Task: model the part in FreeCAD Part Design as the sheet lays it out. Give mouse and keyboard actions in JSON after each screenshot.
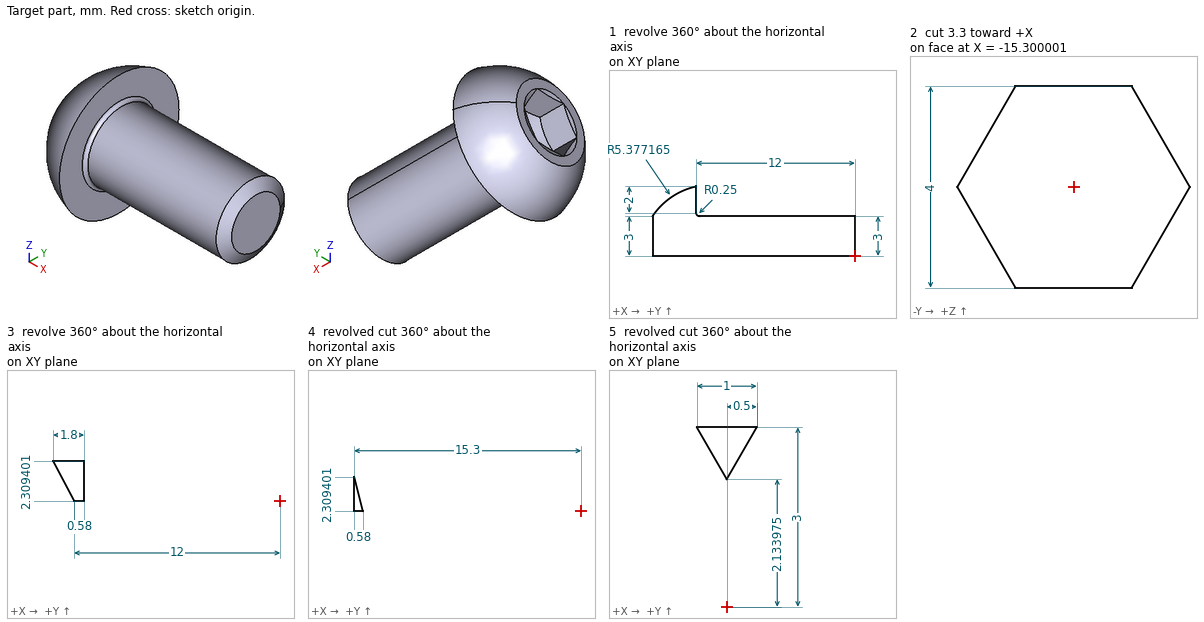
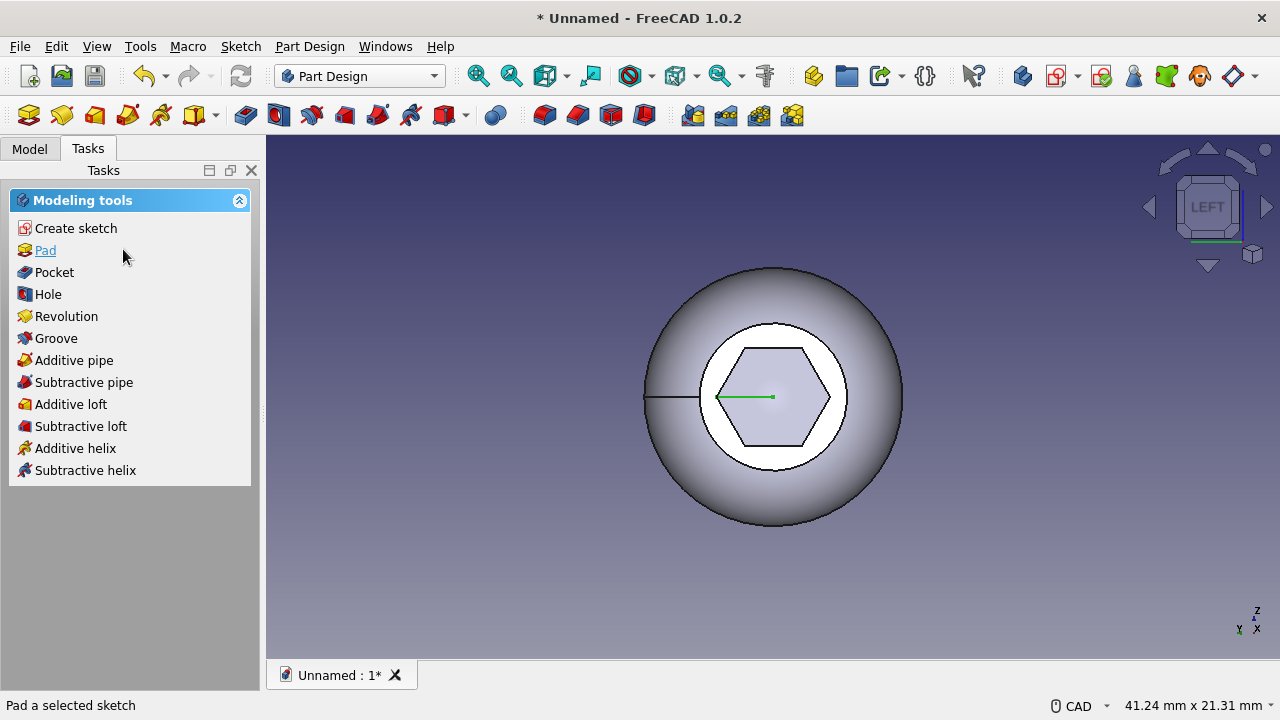
{"action": "left_click", "coordinate": [312, 116]}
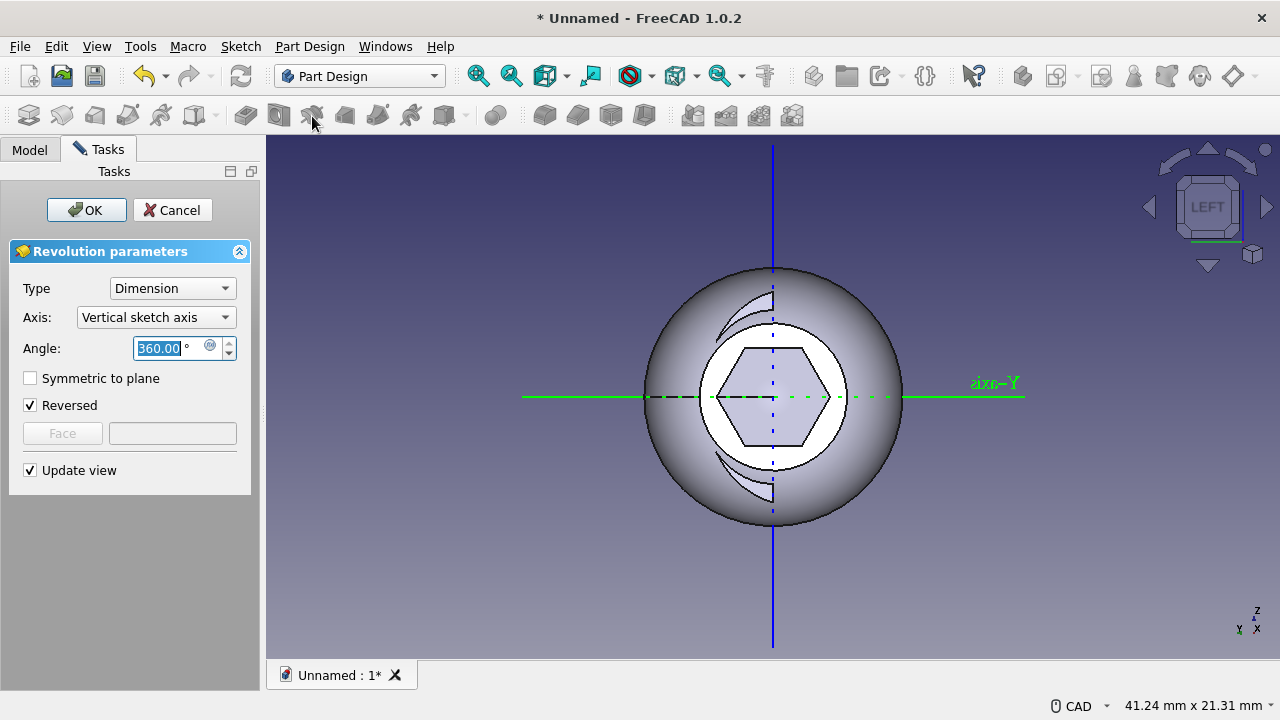
{"action": "left_click", "coordinate": [157, 318]}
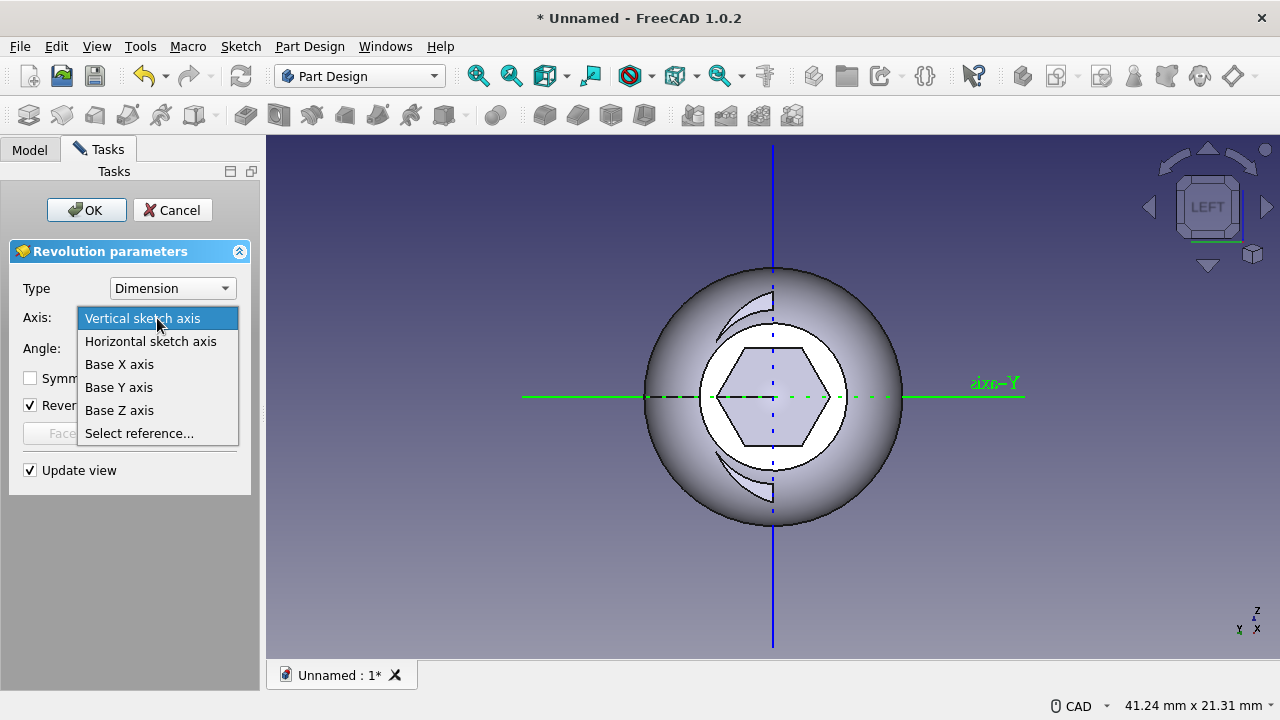
{"action": "left_click", "coordinate": [156, 342]}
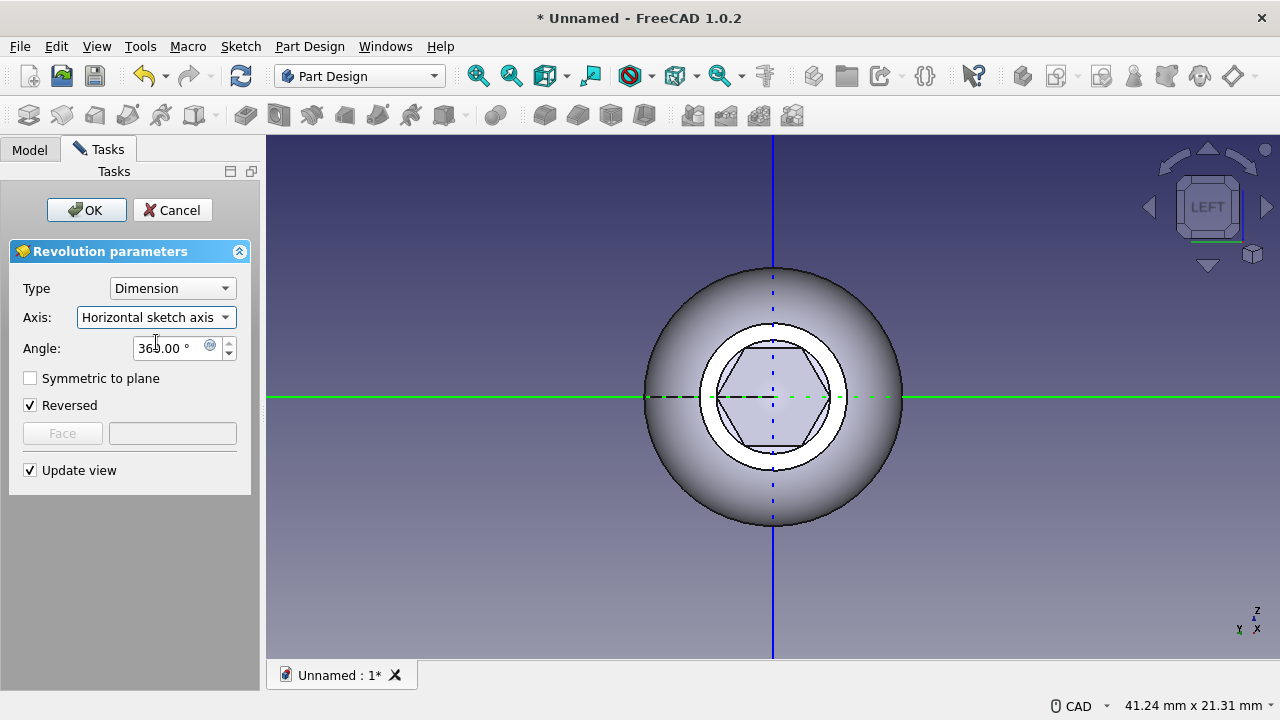
{"action": "left_click", "coordinate": [87, 210]}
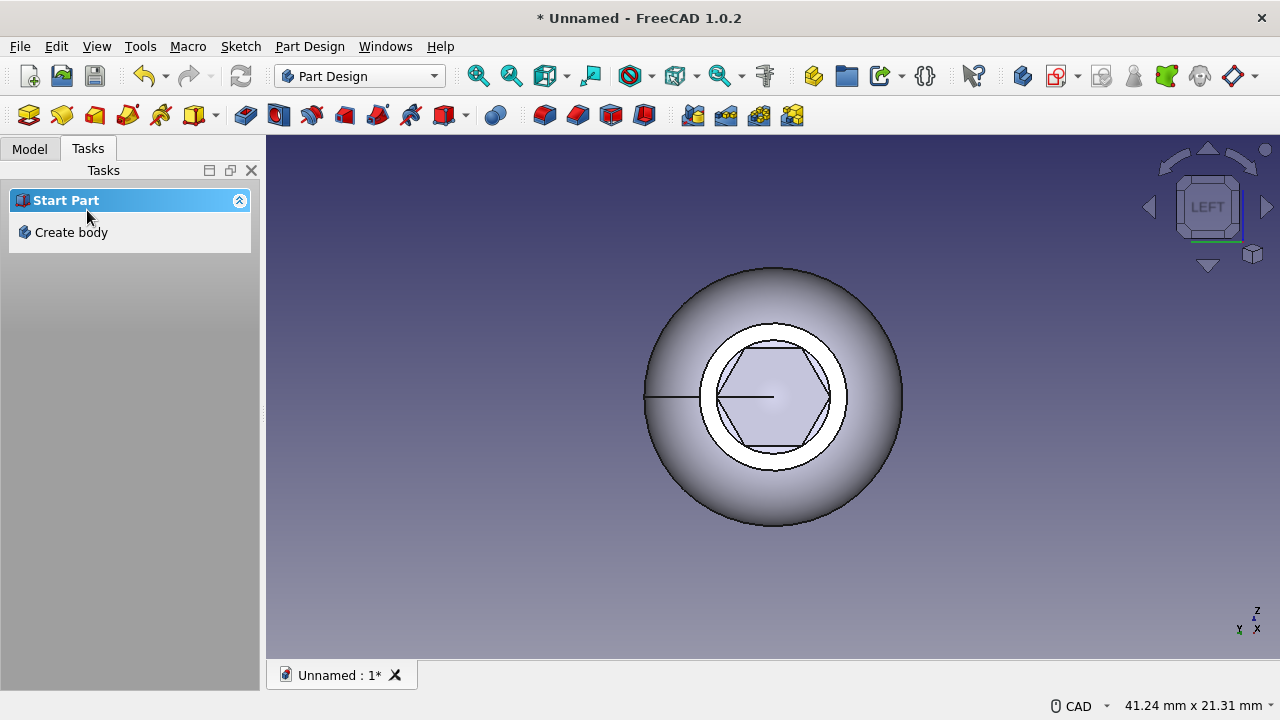
{"action": "left_click", "coordinate": [1056, 76]}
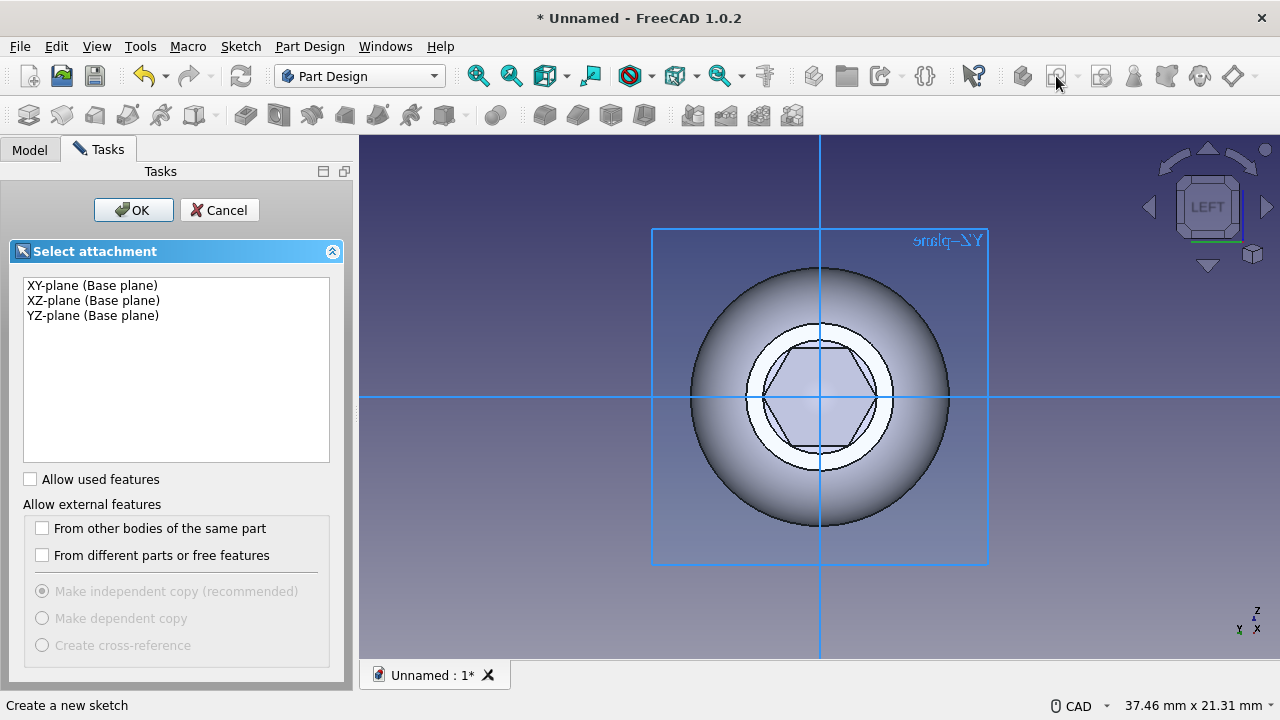
{"action": "left_click", "coordinate": [84, 286]}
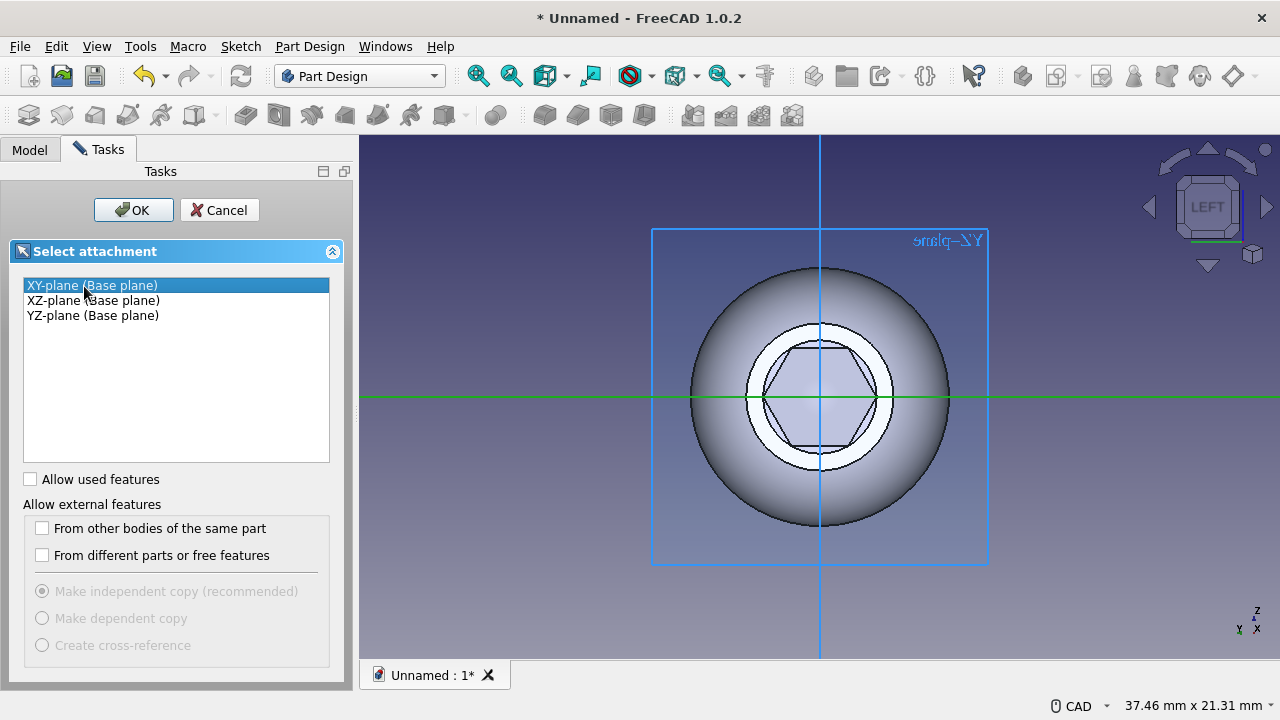
{"action": "left_click", "coordinate": [134, 210]}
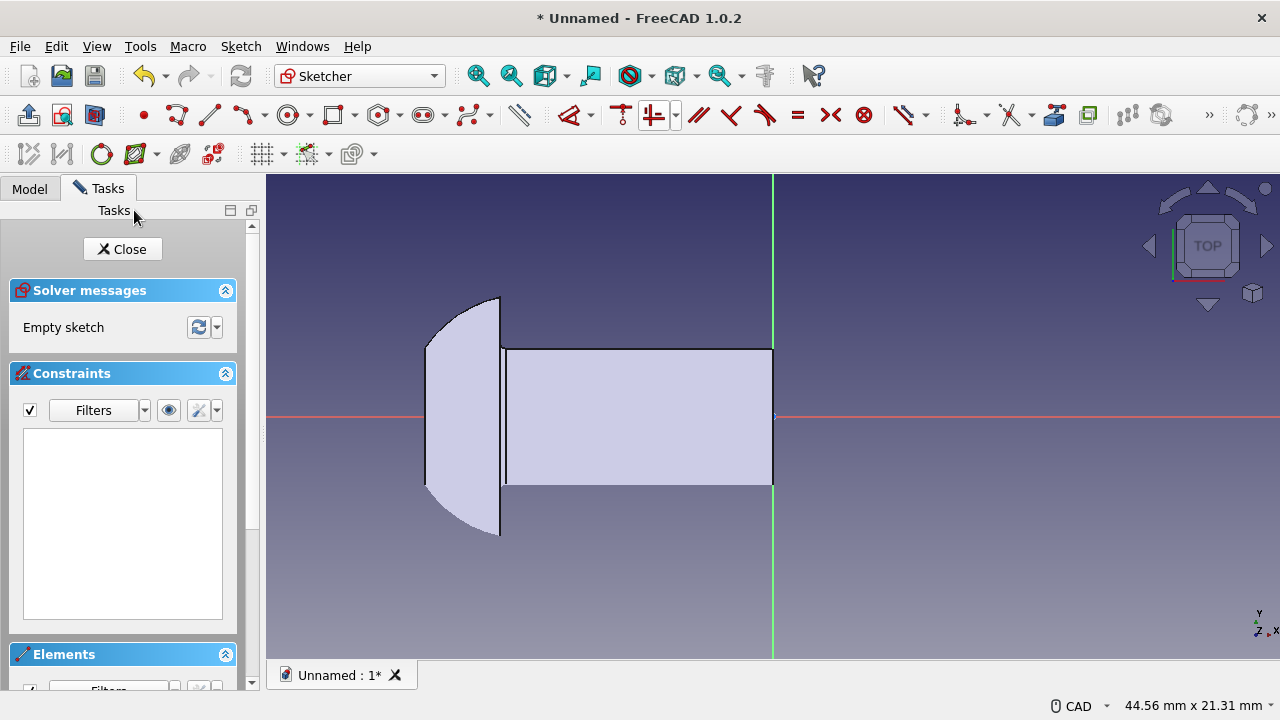
{"action": "left_click", "coordinate": [95, 116]}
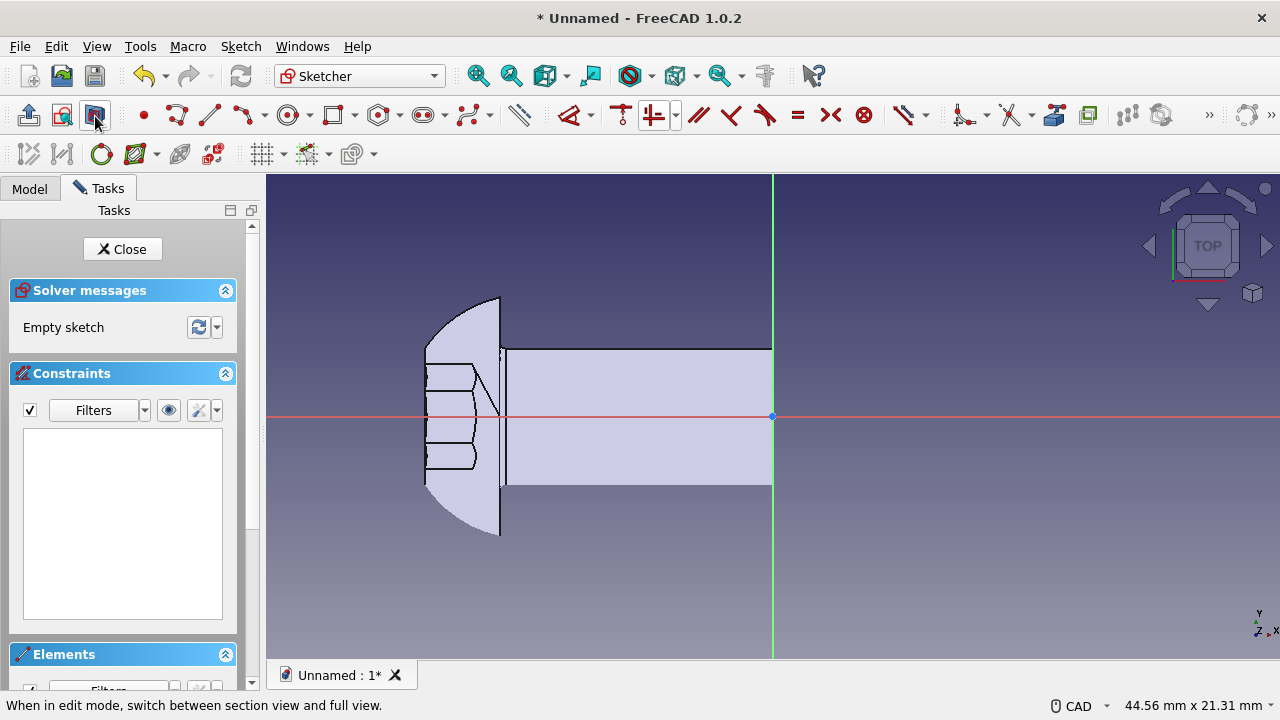
{"action": "scroll", "coordinate": [777, 355], "scroll_direction": "up", "scroll_amount": 14}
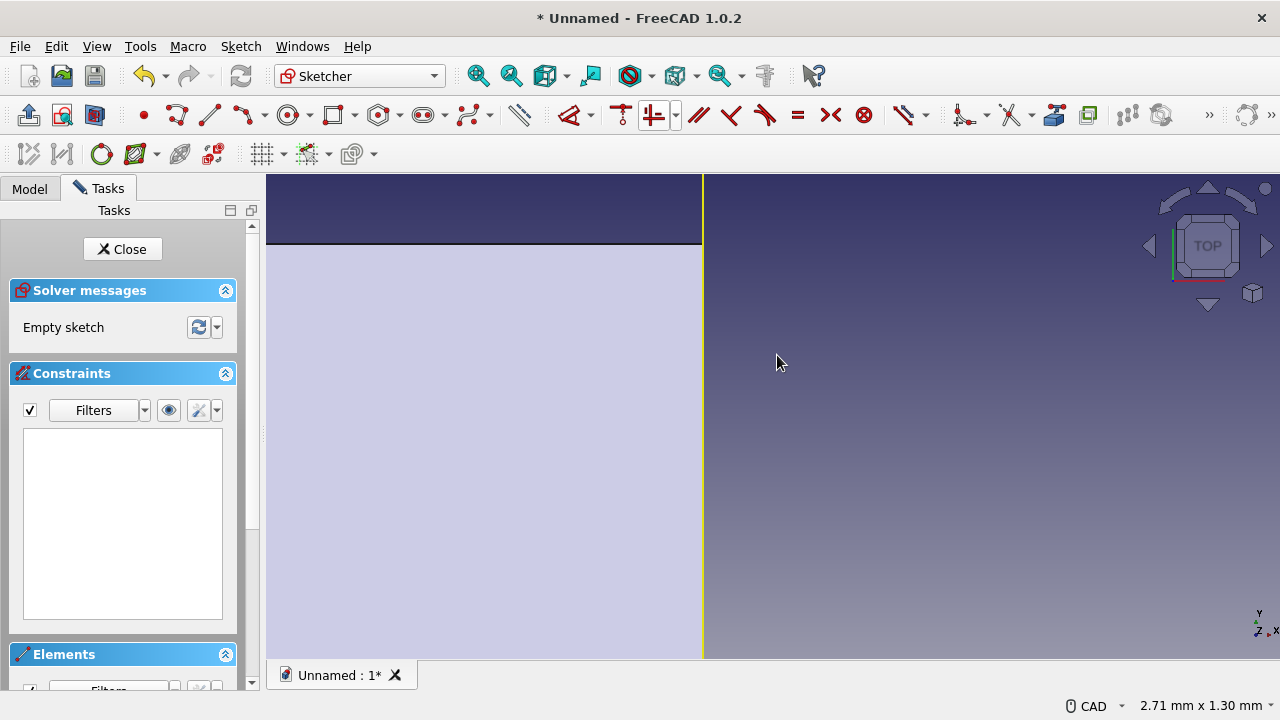
{"action": "left_click", "coordinate": [177, 116]}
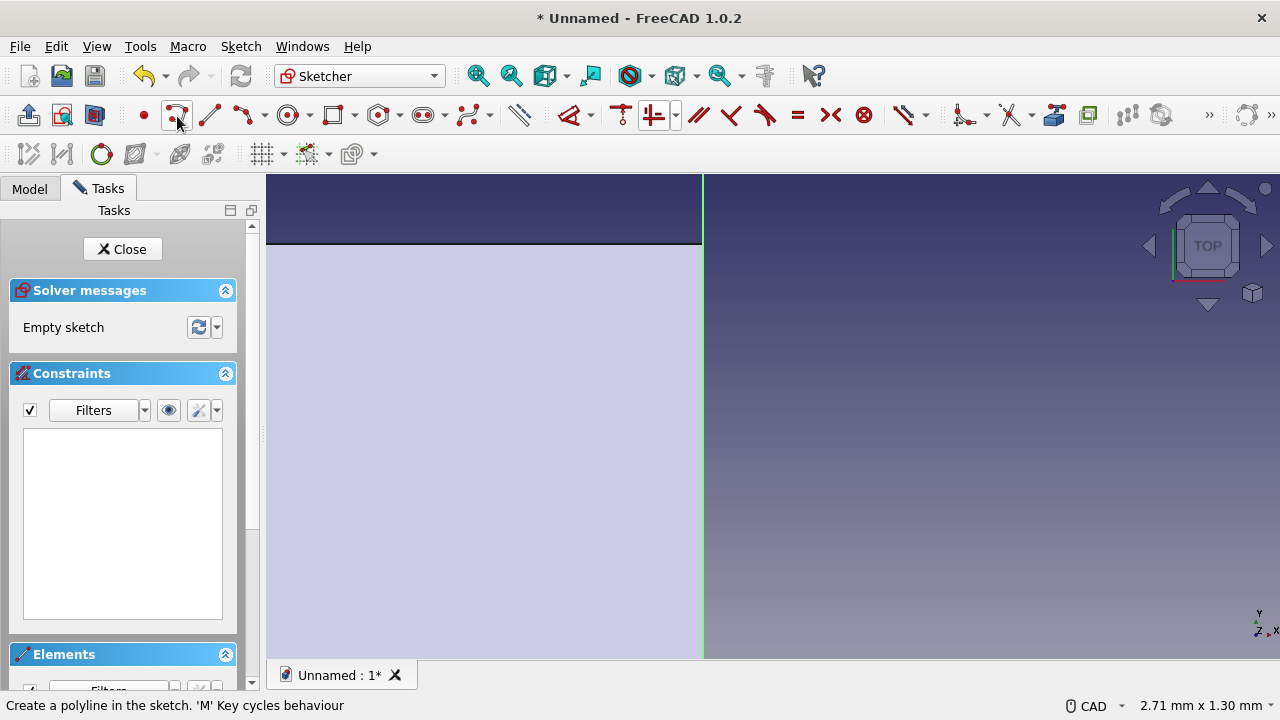
{"action": "left_click", "coordinate": [703, 568]}
{"action": "left_click", "coordinate": [891, 244]}
{"action": "left_click", "coordinate": [516, 244]}
{"action": "left_click", "coordinate": [703, 569]}
{"action": "key", "text": "Escape"}
{"action": "key", "text": "Escape"}